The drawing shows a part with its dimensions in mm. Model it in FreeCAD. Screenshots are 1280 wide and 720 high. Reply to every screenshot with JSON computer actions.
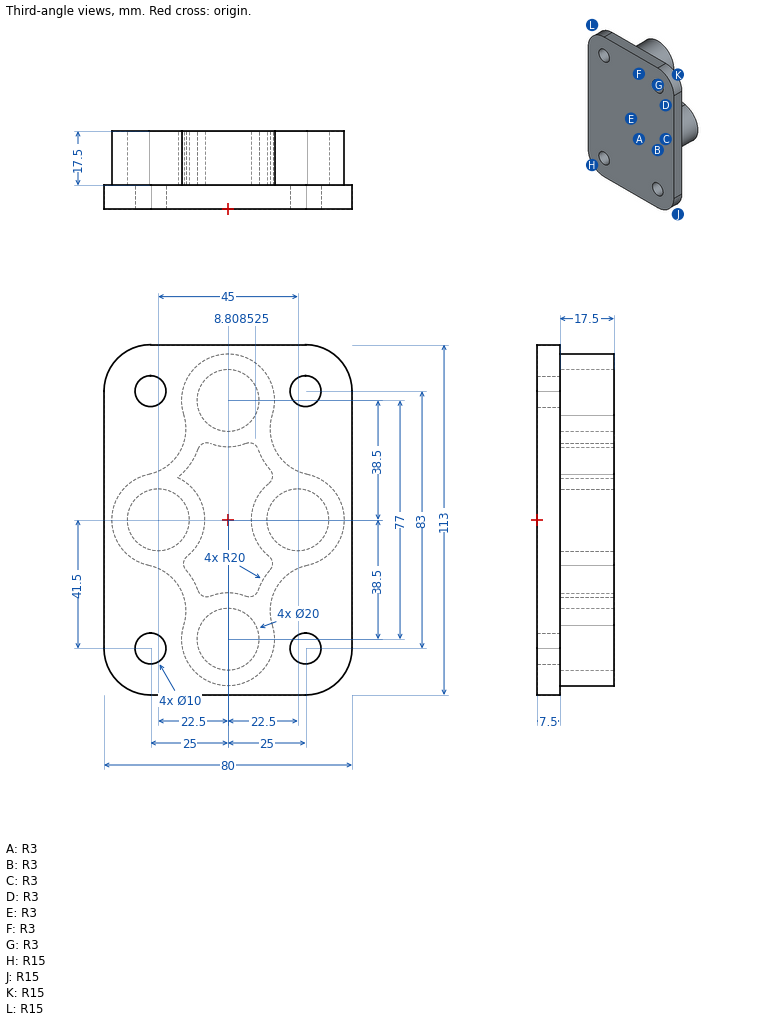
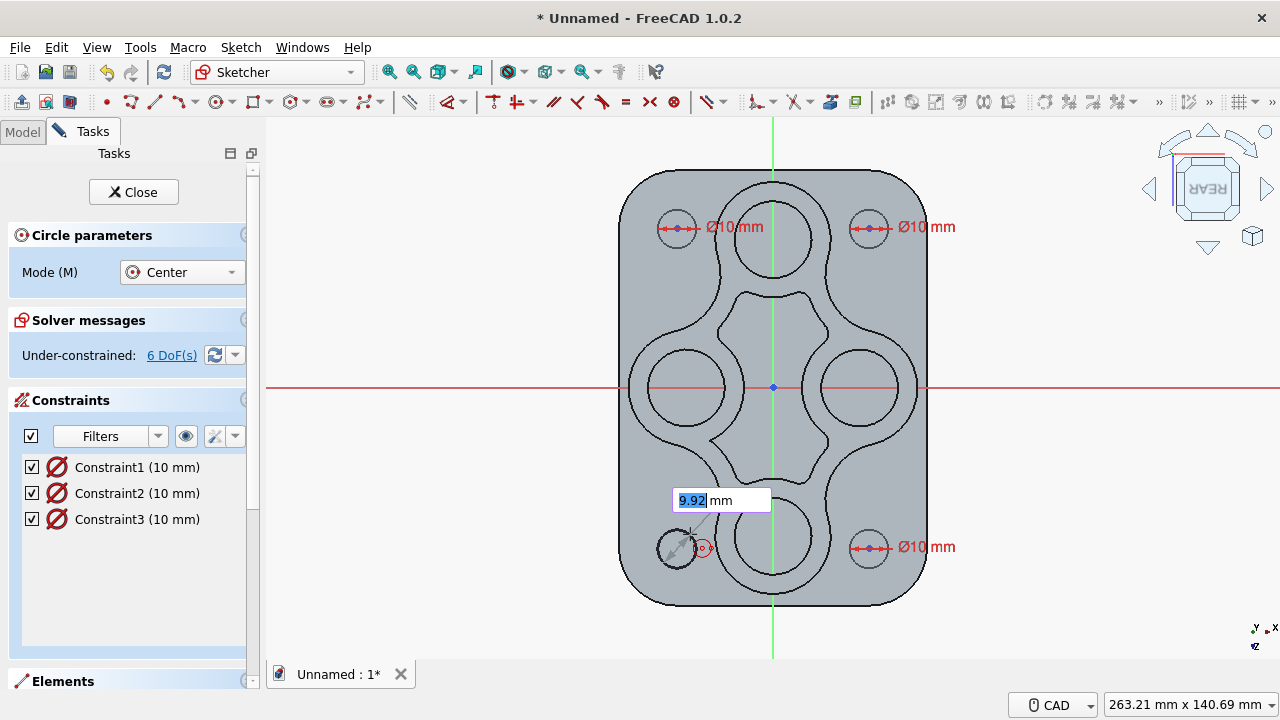
{"action": "type", "text": "10"}
{"action": "key", "text": "Return"}
{"action": "key", "text": "Escape"}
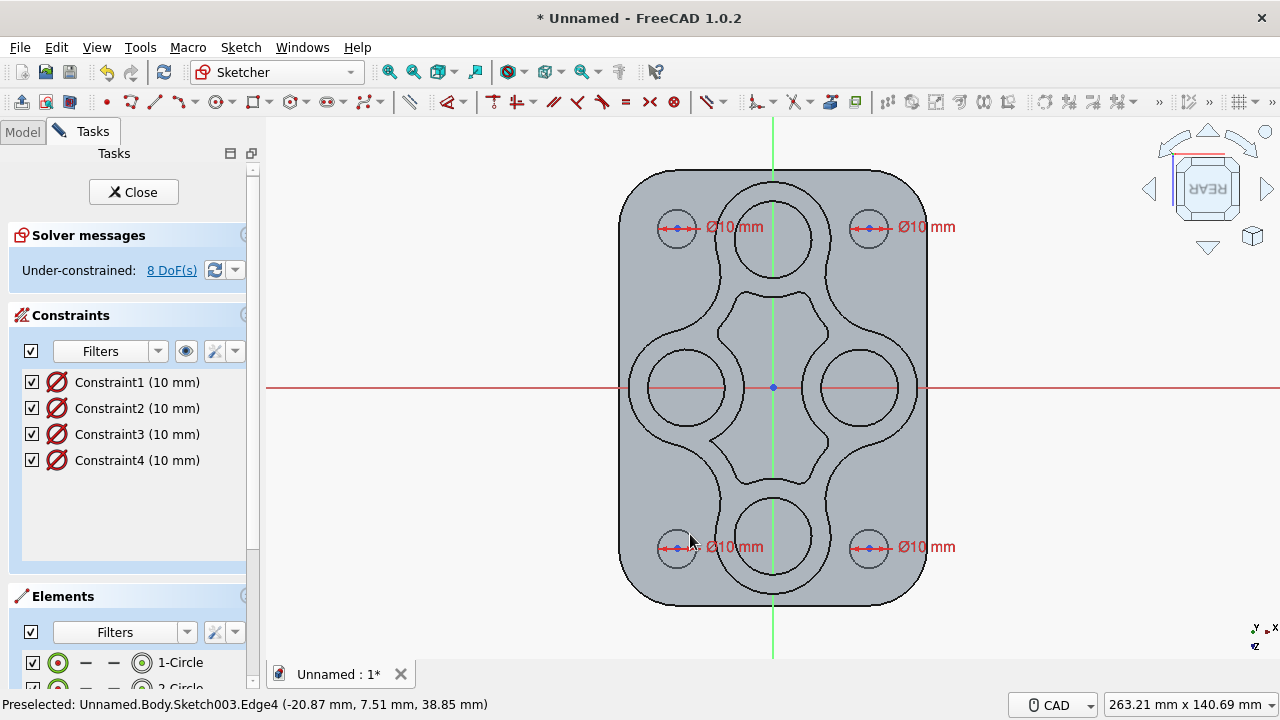
{"action": "left_click", "coordinate": [677, 229]}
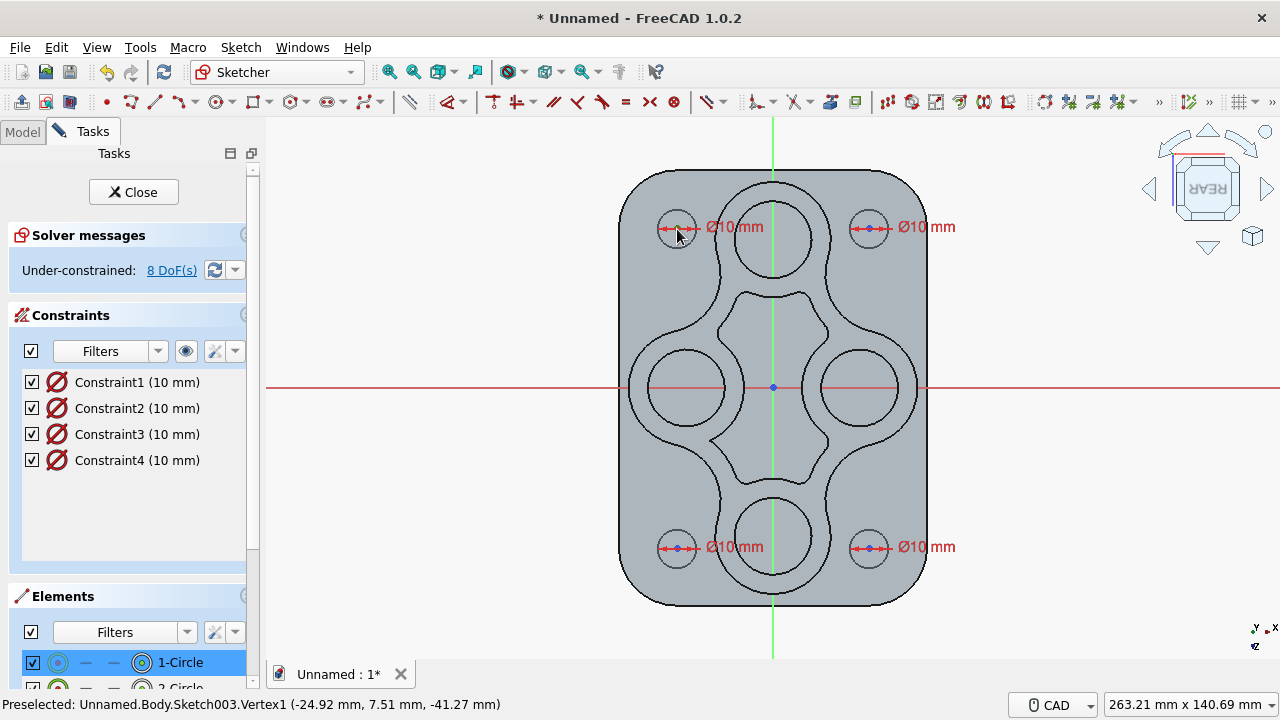
{"action": "left_click", "coordinate": [869, 229]}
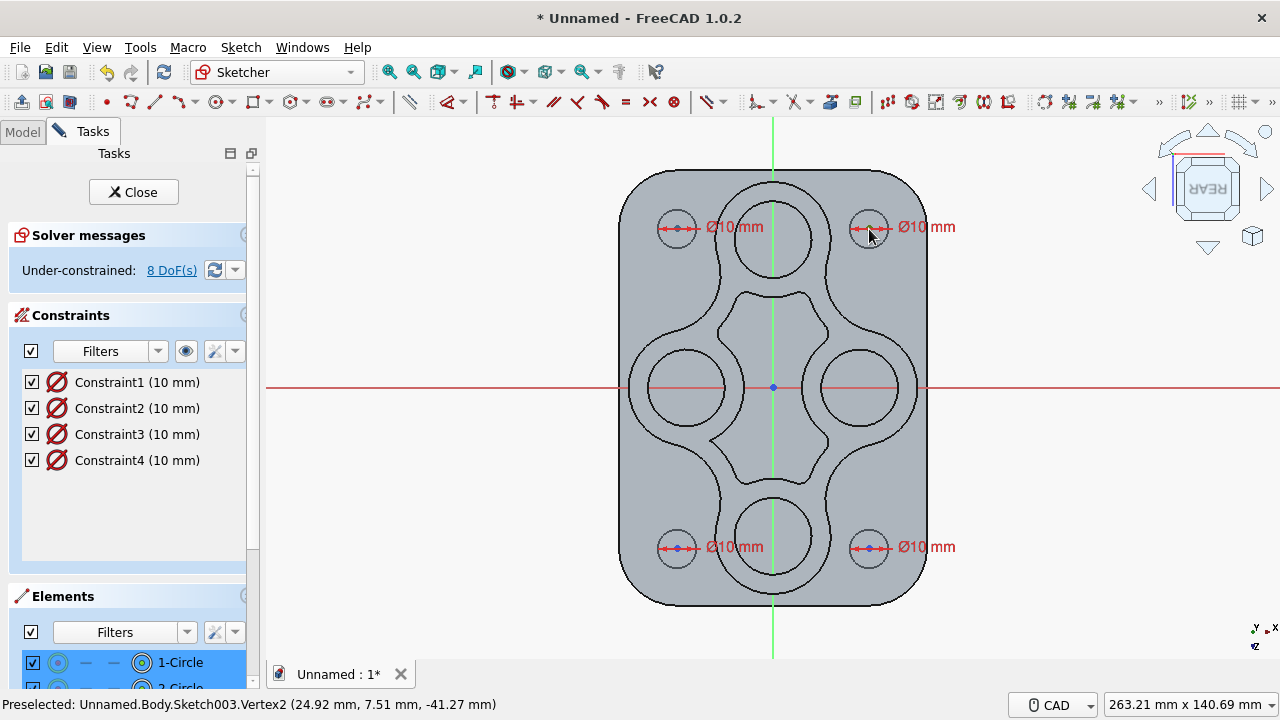
{"action": "key", "text": "h"}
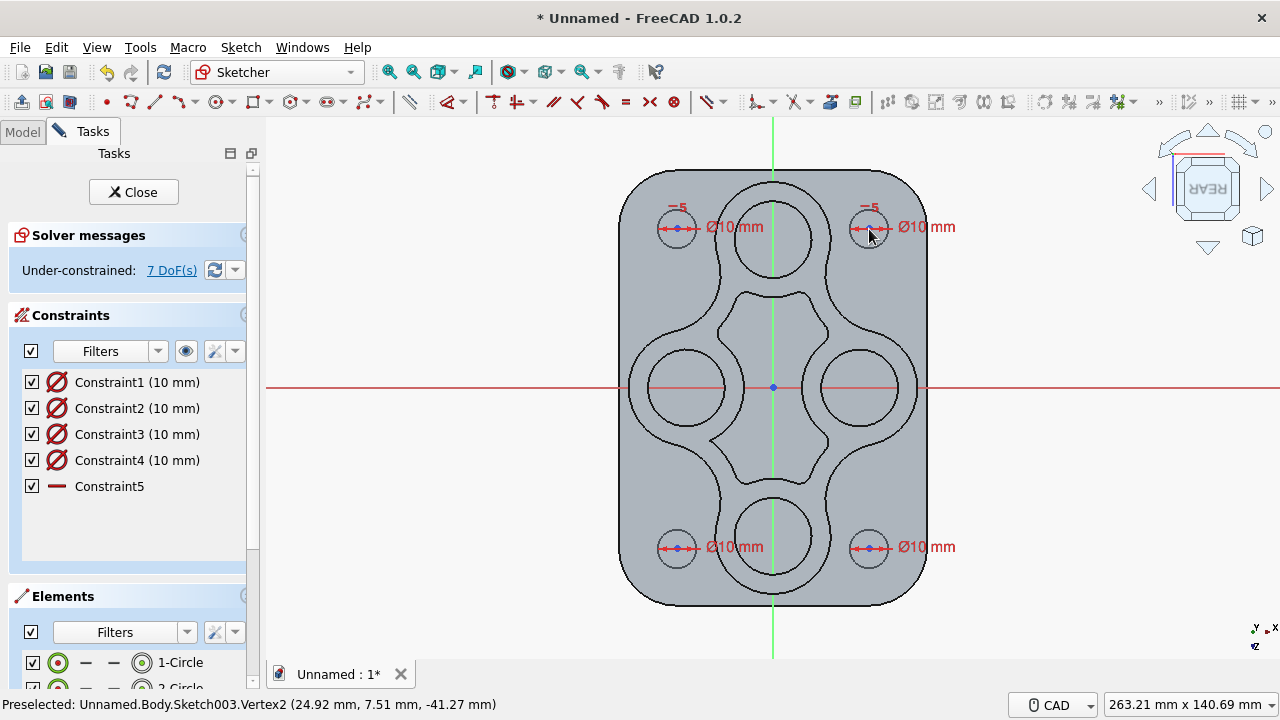
{"action": "left_click", "coordinate": [869, 229]}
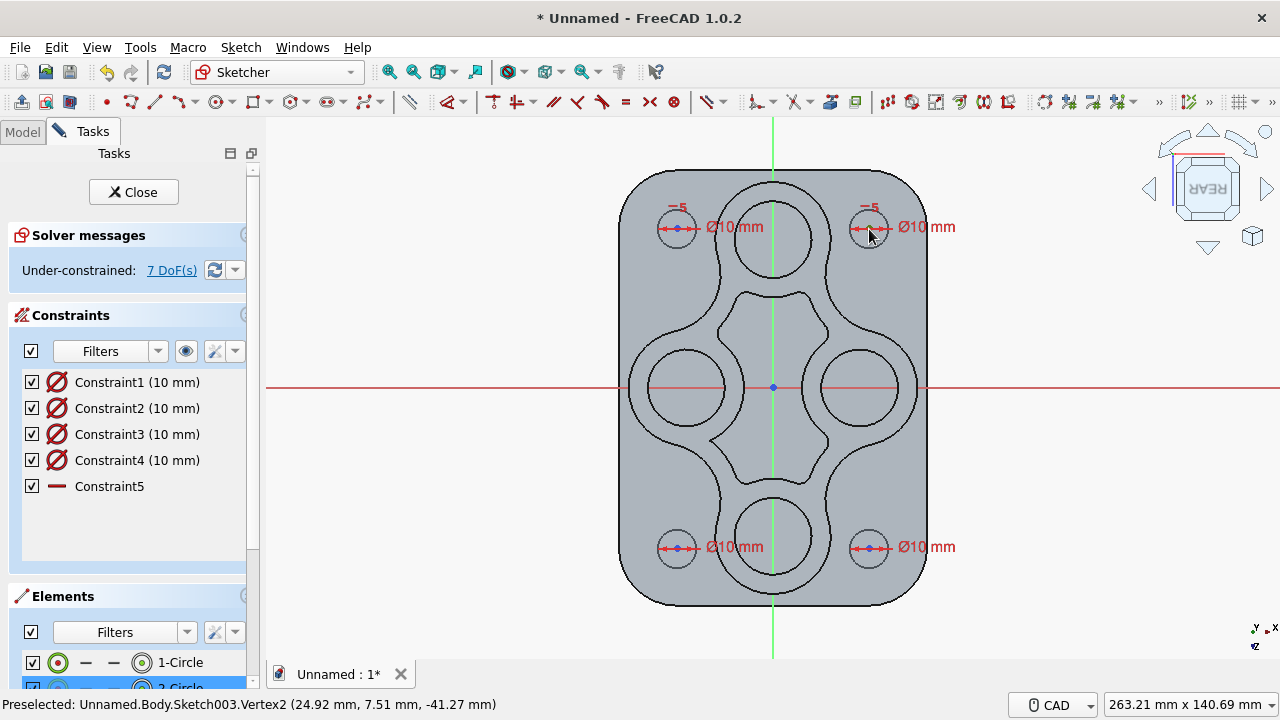
{"action": "left_click", "coordinate": [869, 549]}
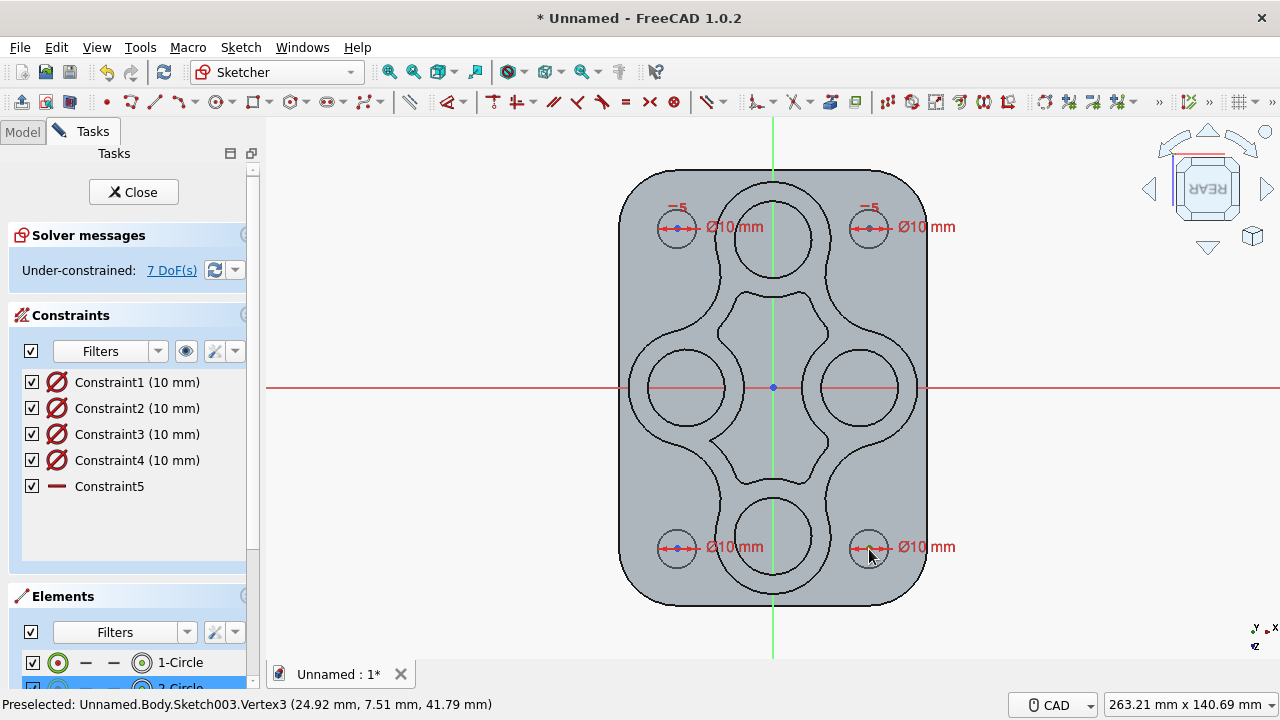
{"action": "key", "text": "v"}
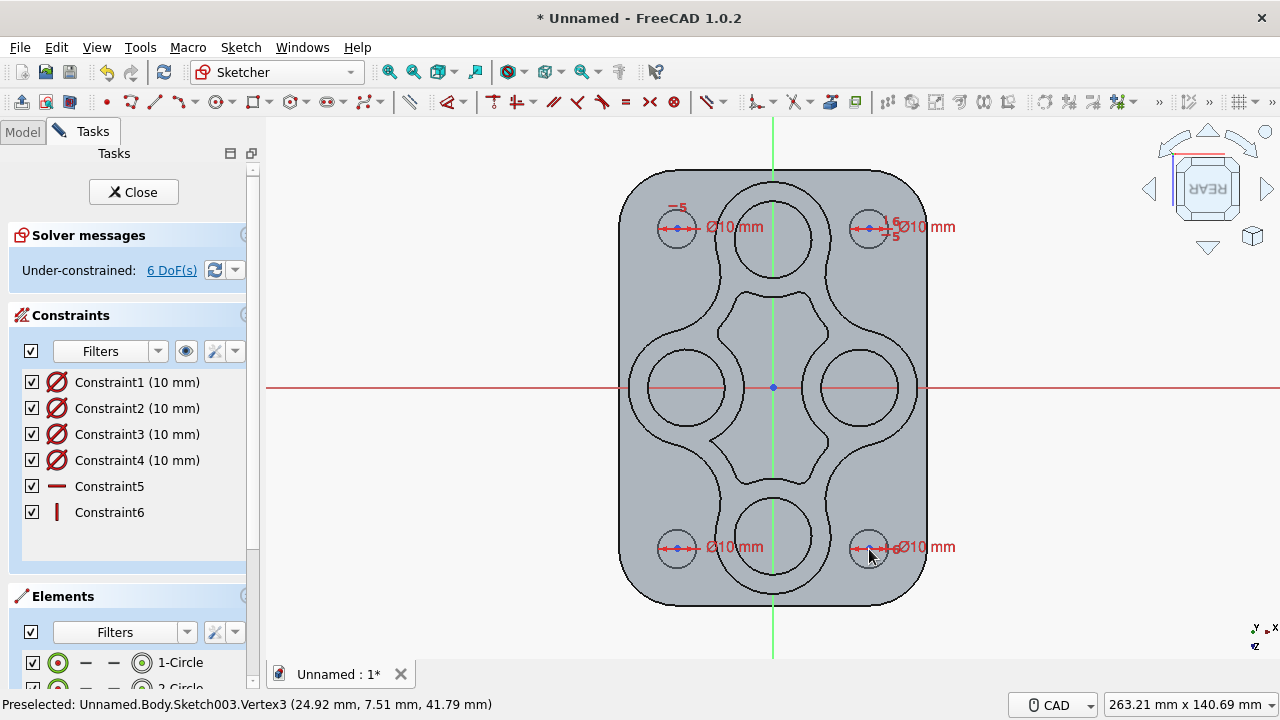
{"action": "left_click", "coordinate": [677, 229]}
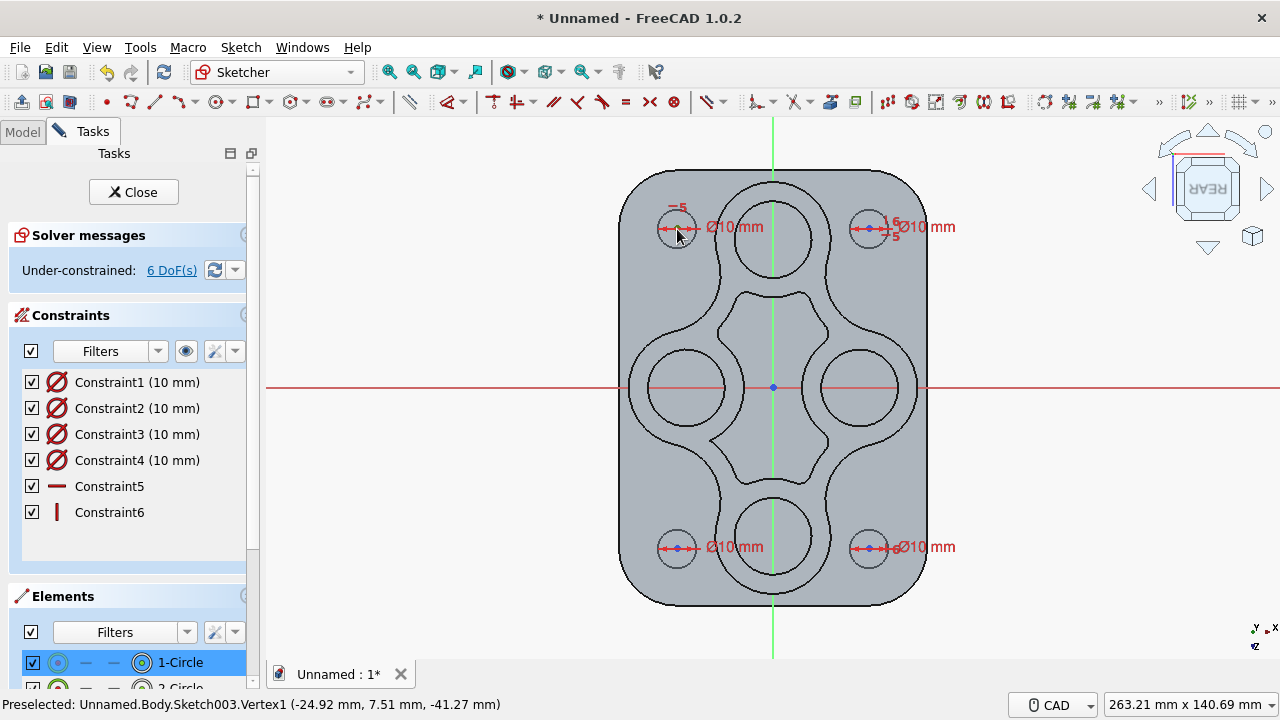
{"action": "left_click", "coordinate": [677, 549]}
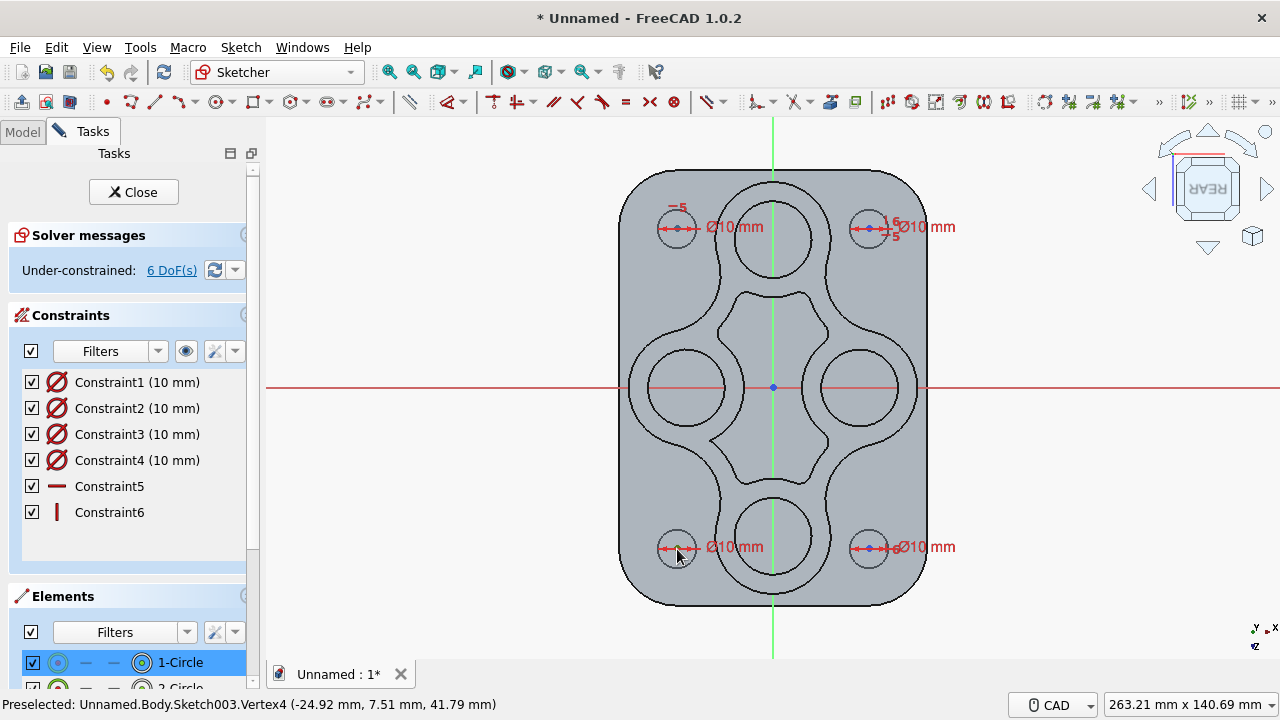
{"action": "key", "text": "v"}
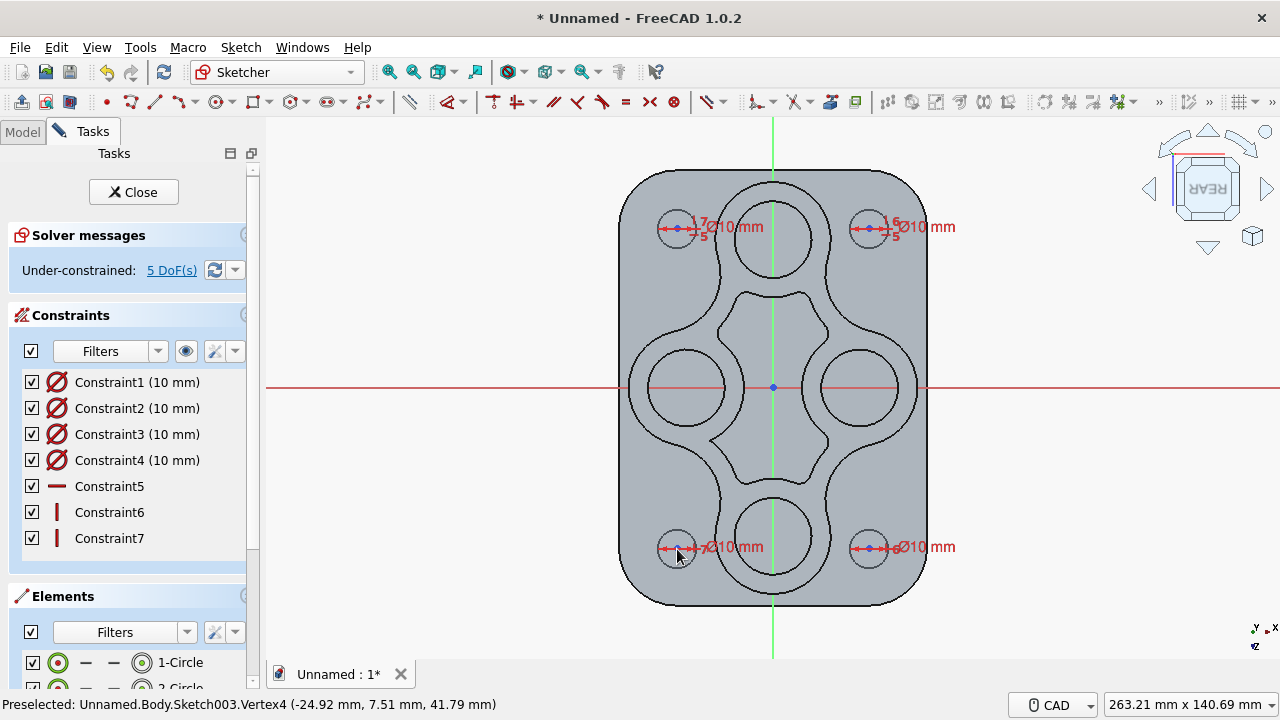
{"action": "left_click", "coordinate": [869, 549]}